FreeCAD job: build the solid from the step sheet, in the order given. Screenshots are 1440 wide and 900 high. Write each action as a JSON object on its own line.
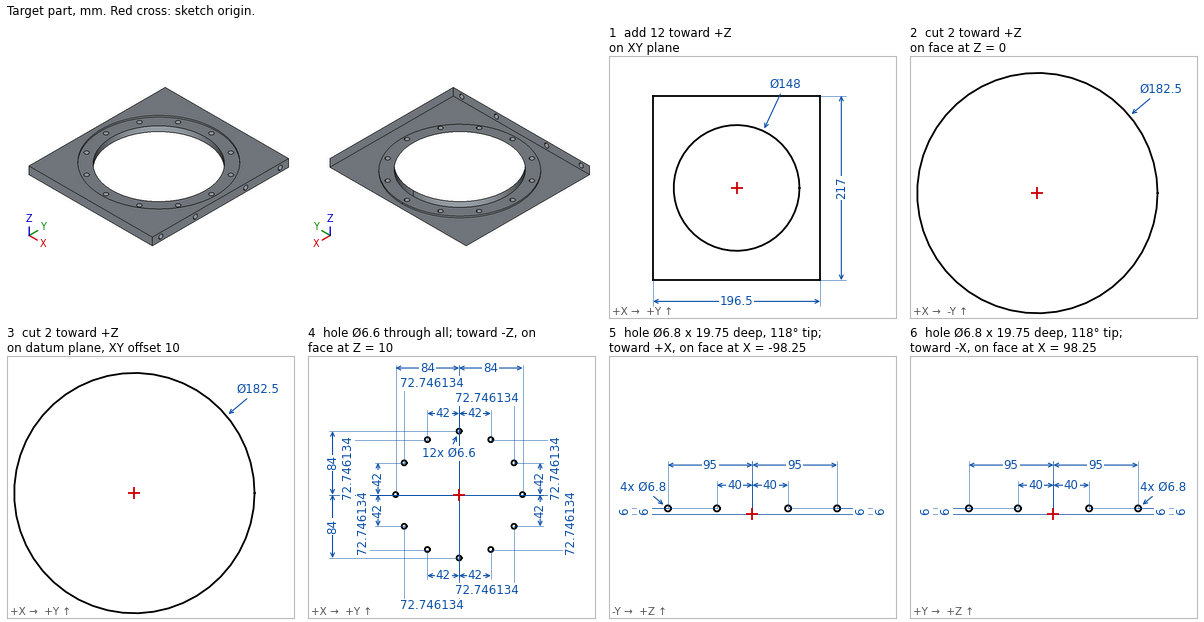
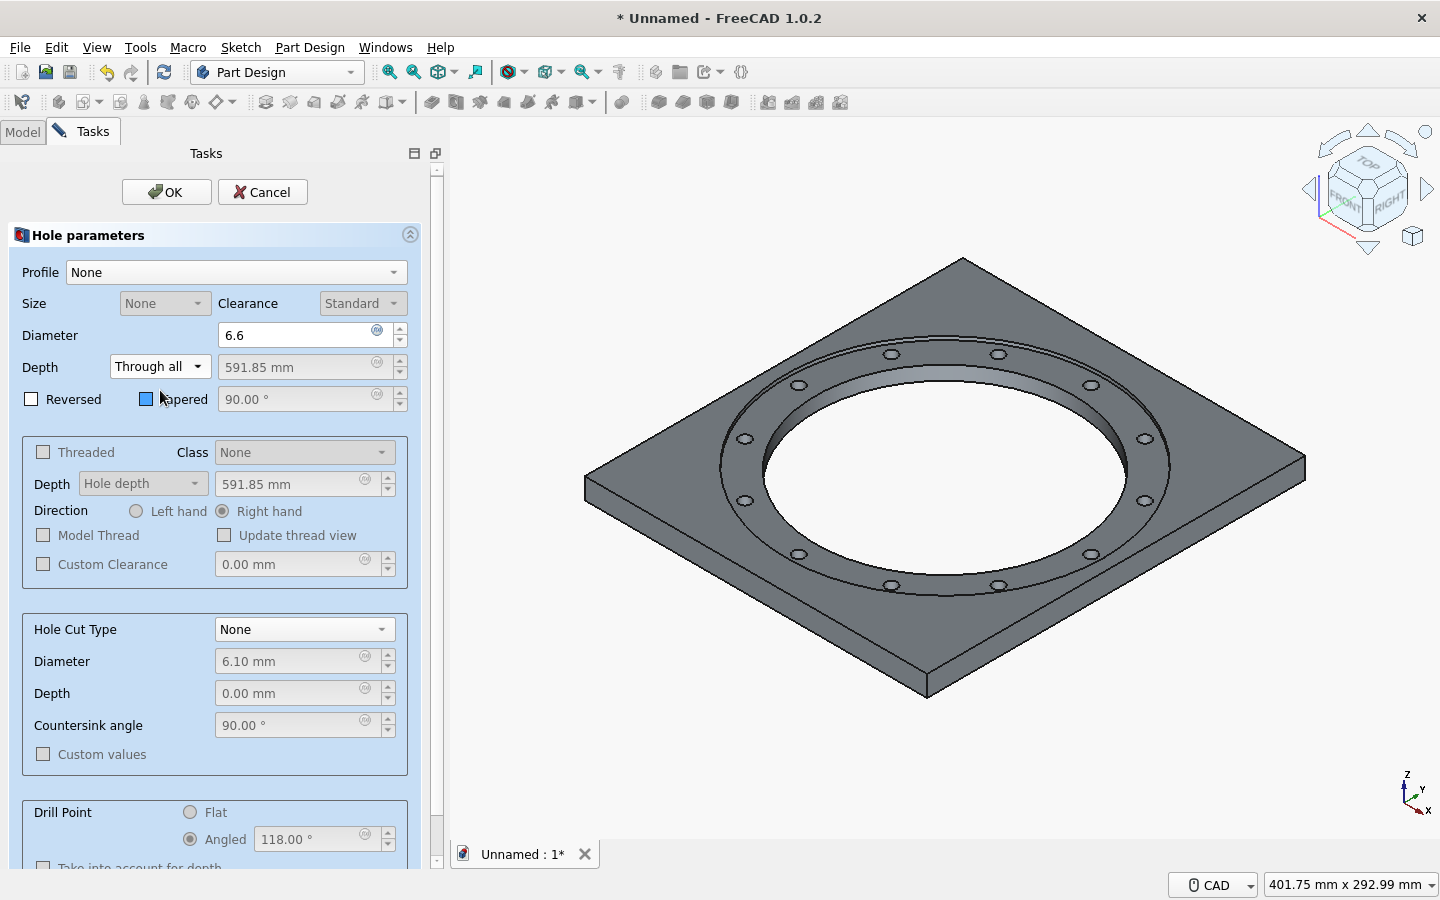
{"action": "left_click", "coordinate": [167, 192]}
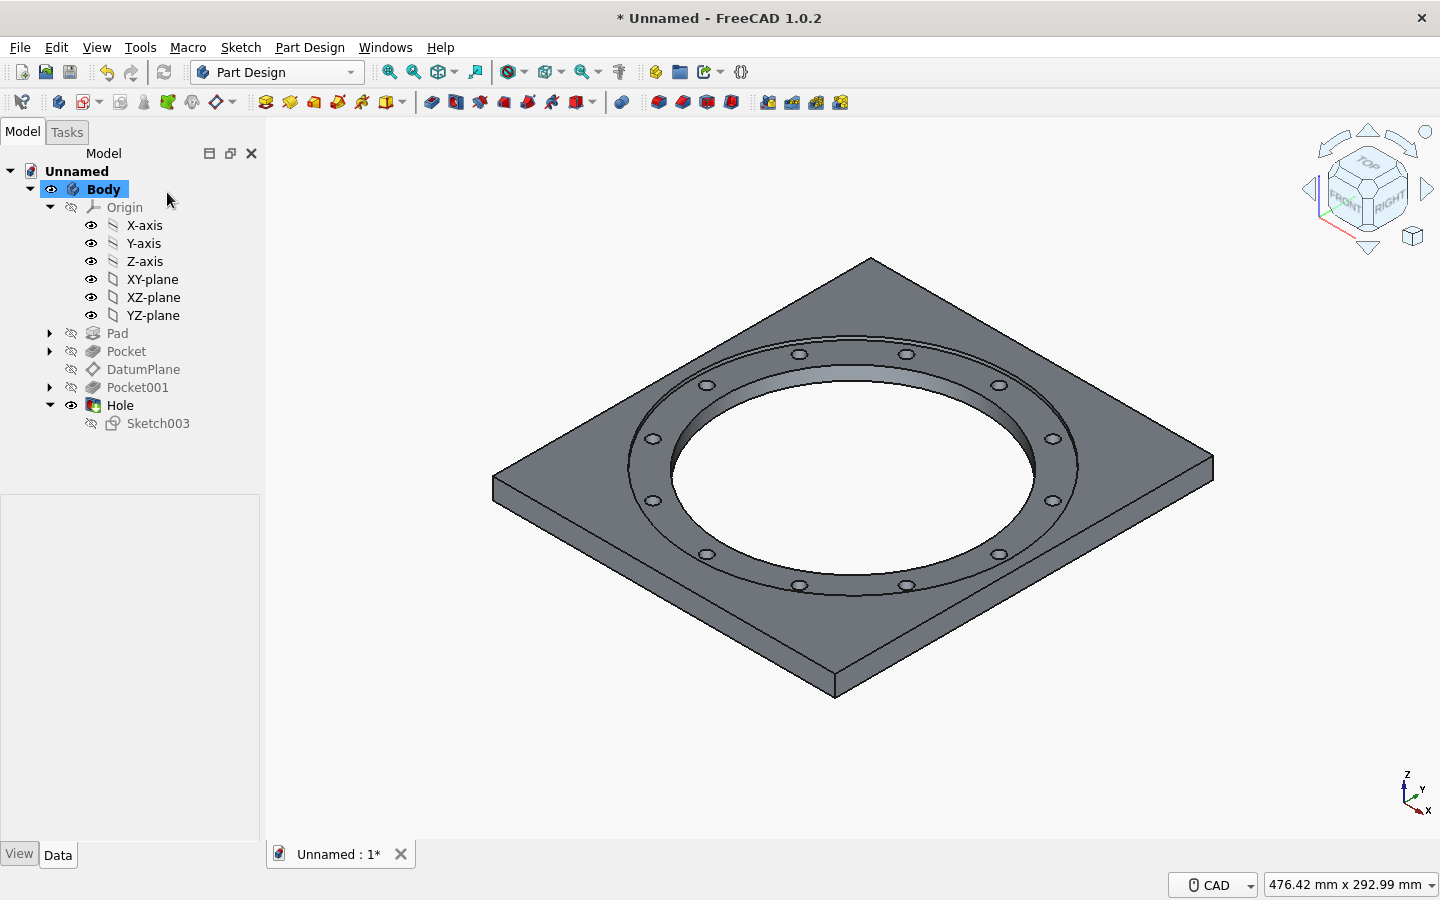
{"action": "key", "text": "6"}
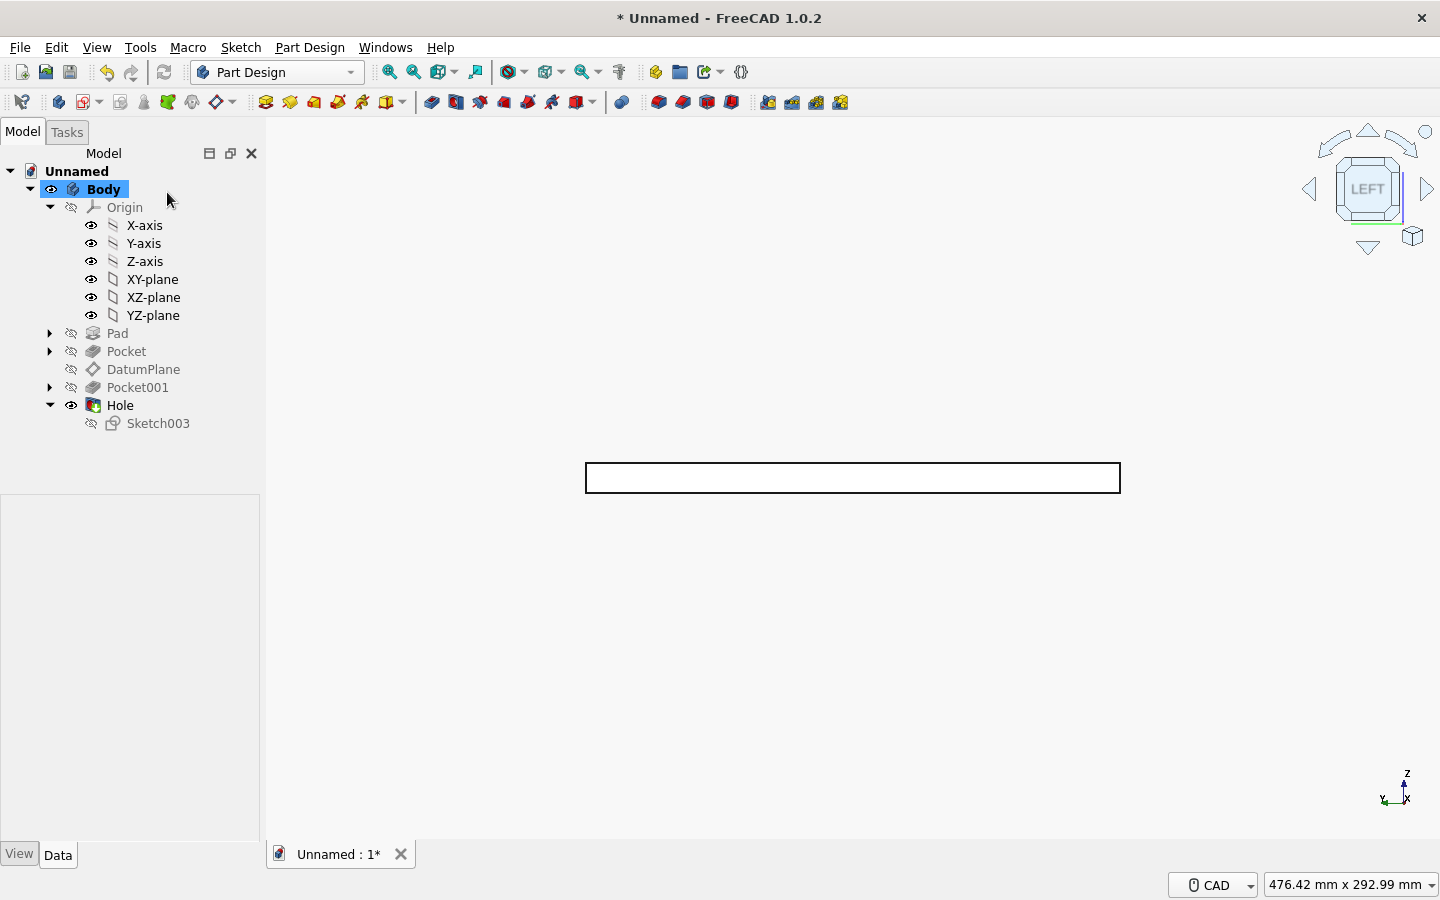
{"action": "left_click", "coordinate": [624, 477]}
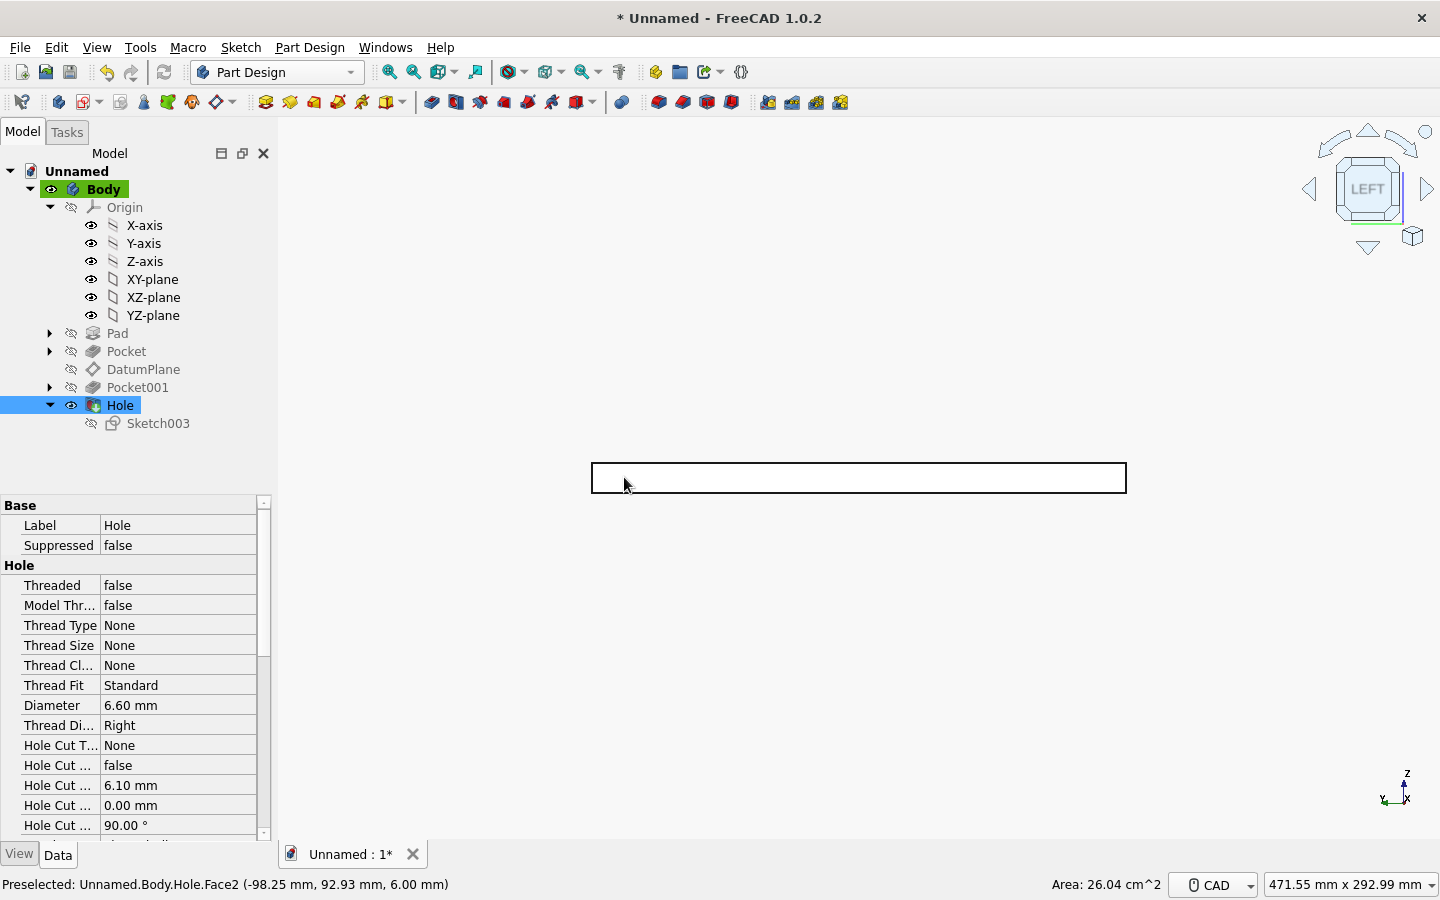
{"action": "left_click", "coordinate": [84, 102]}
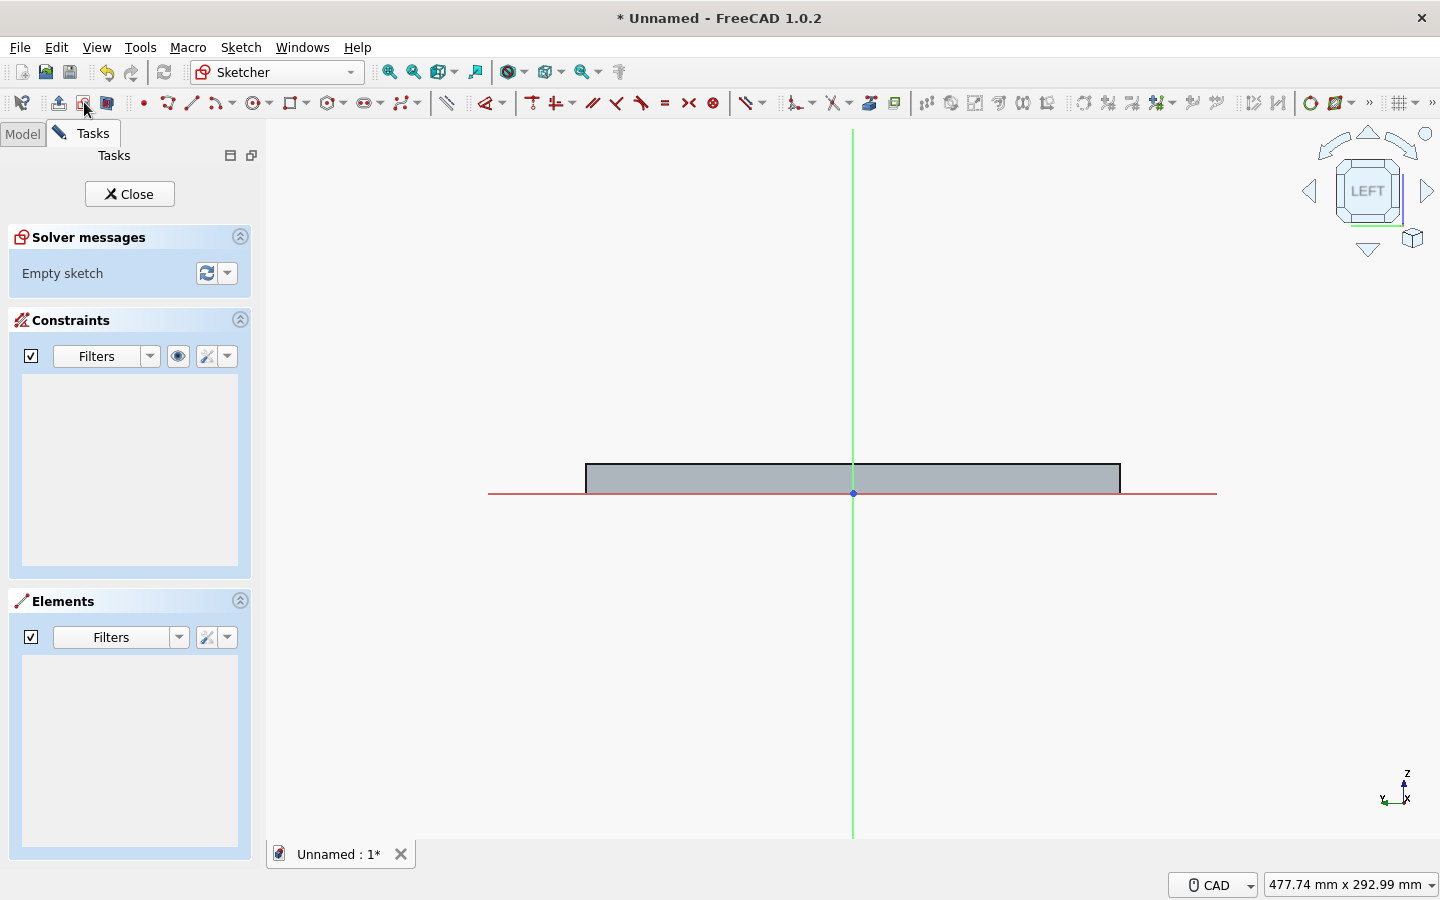
{"action": "scroll", "coordinate": [992, 489], "scroll_direction": "up", "scroll_amount": 2}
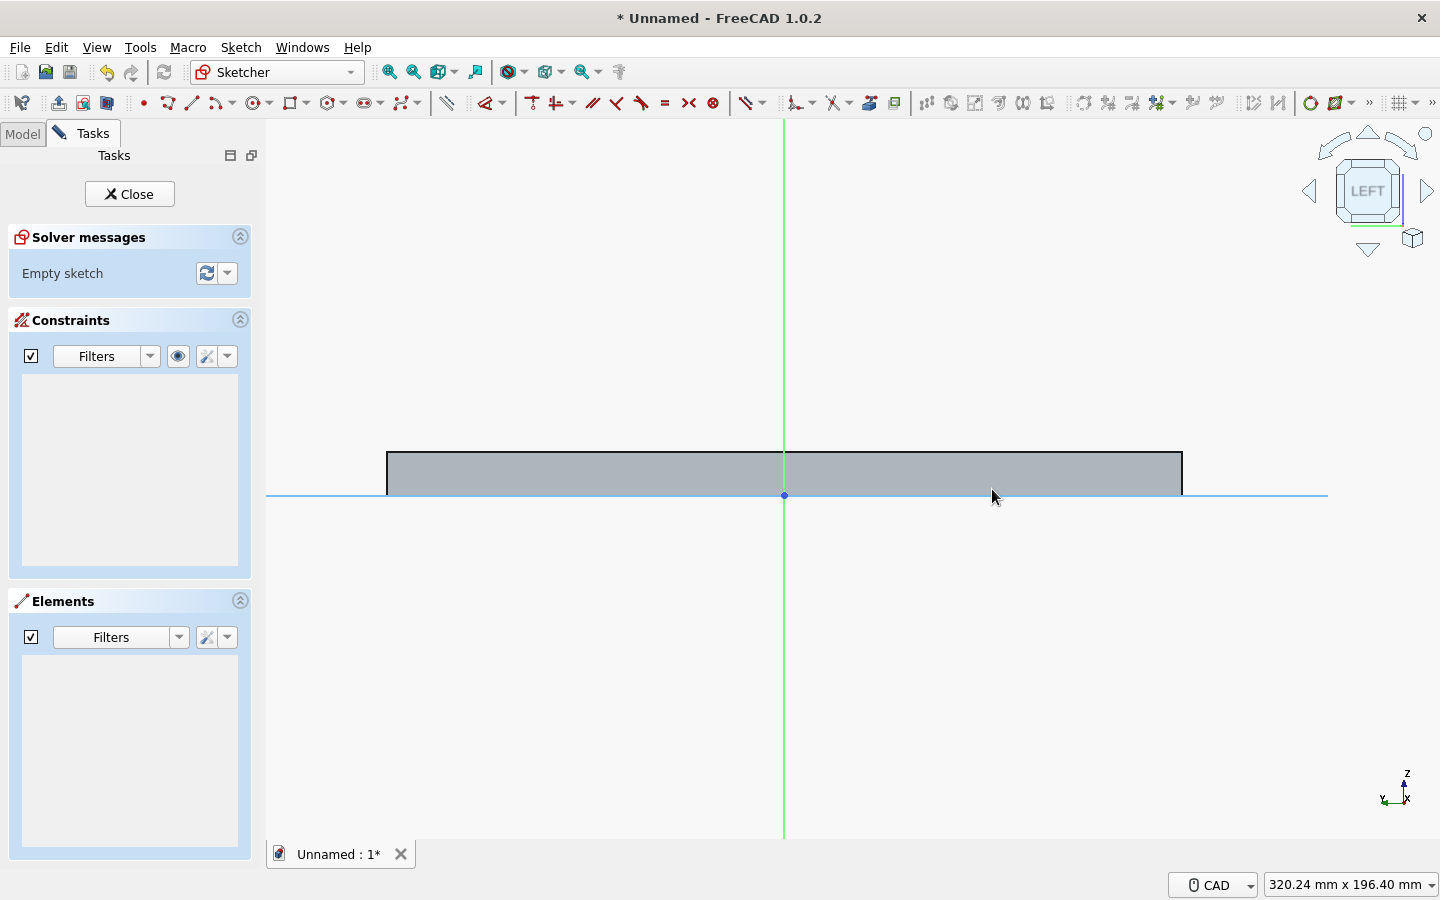
{"action": "left_click", "coordinate": [254, 104]}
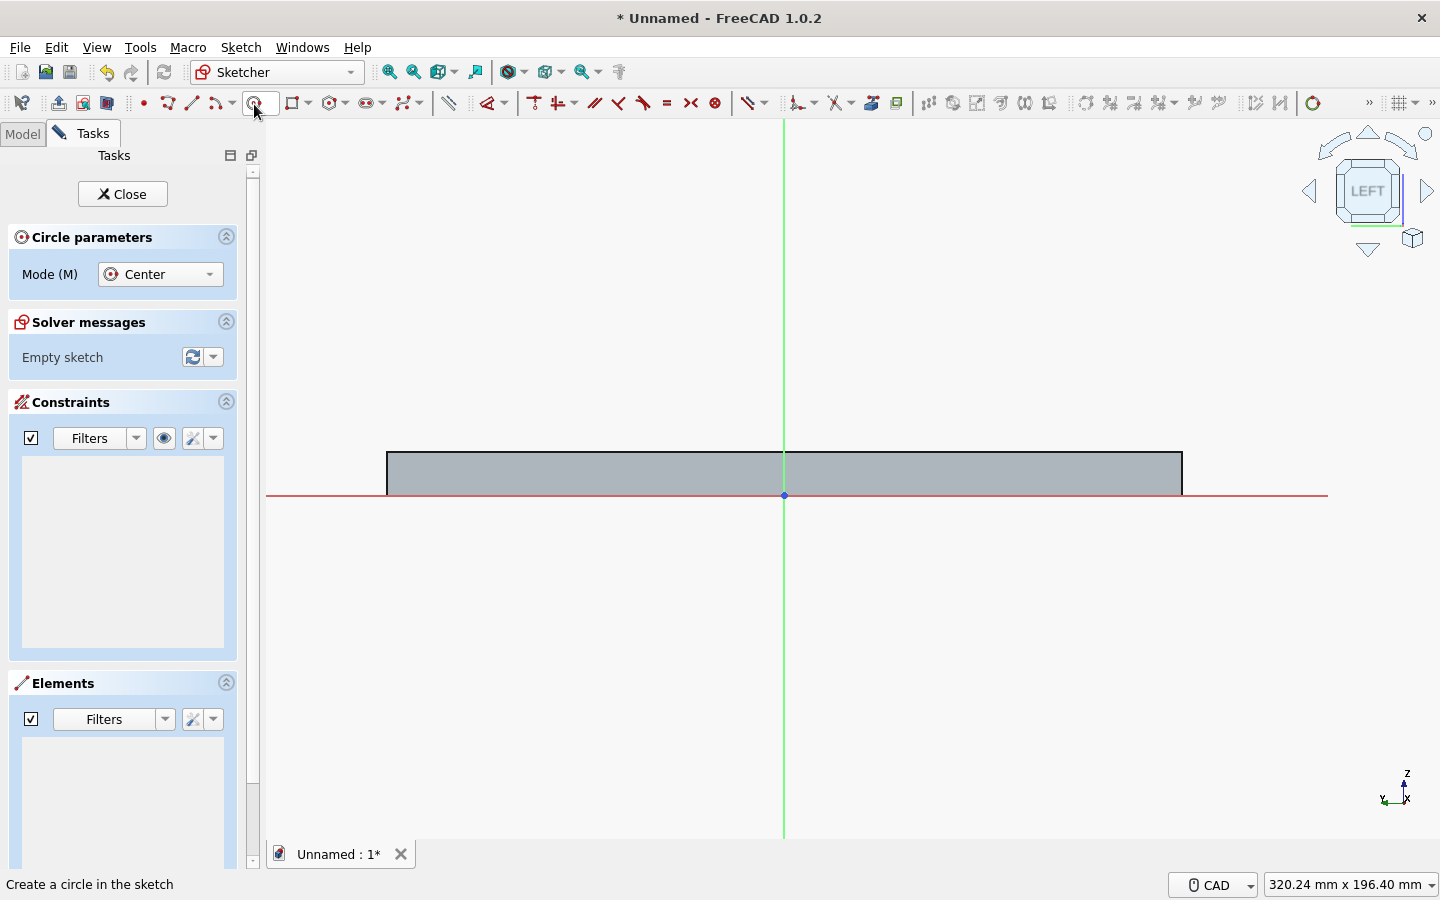
{"action": "scroll", "coordinate": [436, 474], "scroll_direction": "up", "scroll_amount": 3}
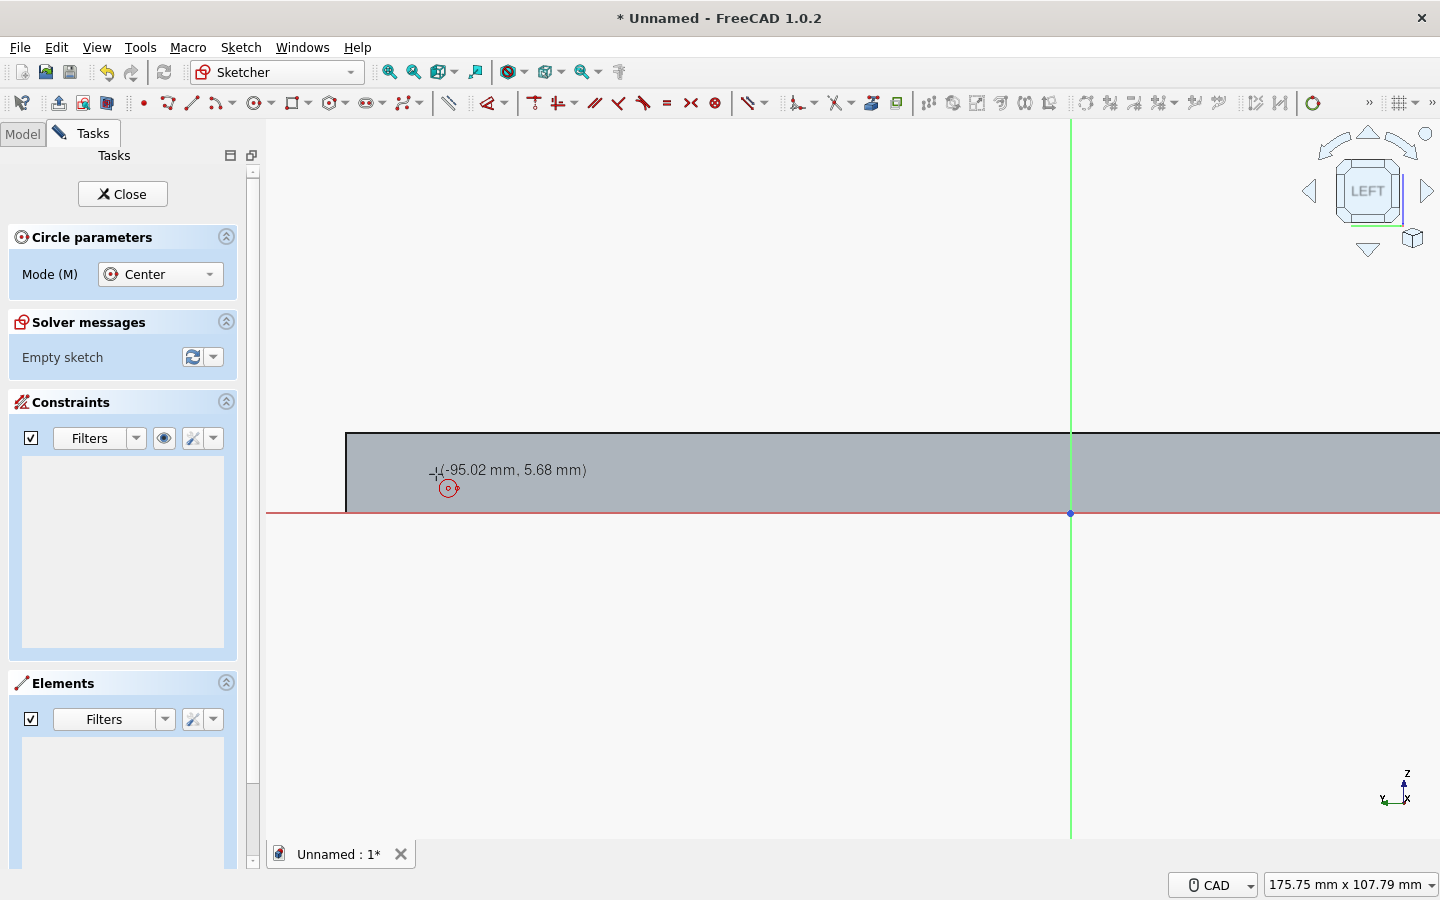
{"action": "left_click", "coordinate": [436, 473]}
{"action": "mouse_move", "coordinate": [452, 457]}